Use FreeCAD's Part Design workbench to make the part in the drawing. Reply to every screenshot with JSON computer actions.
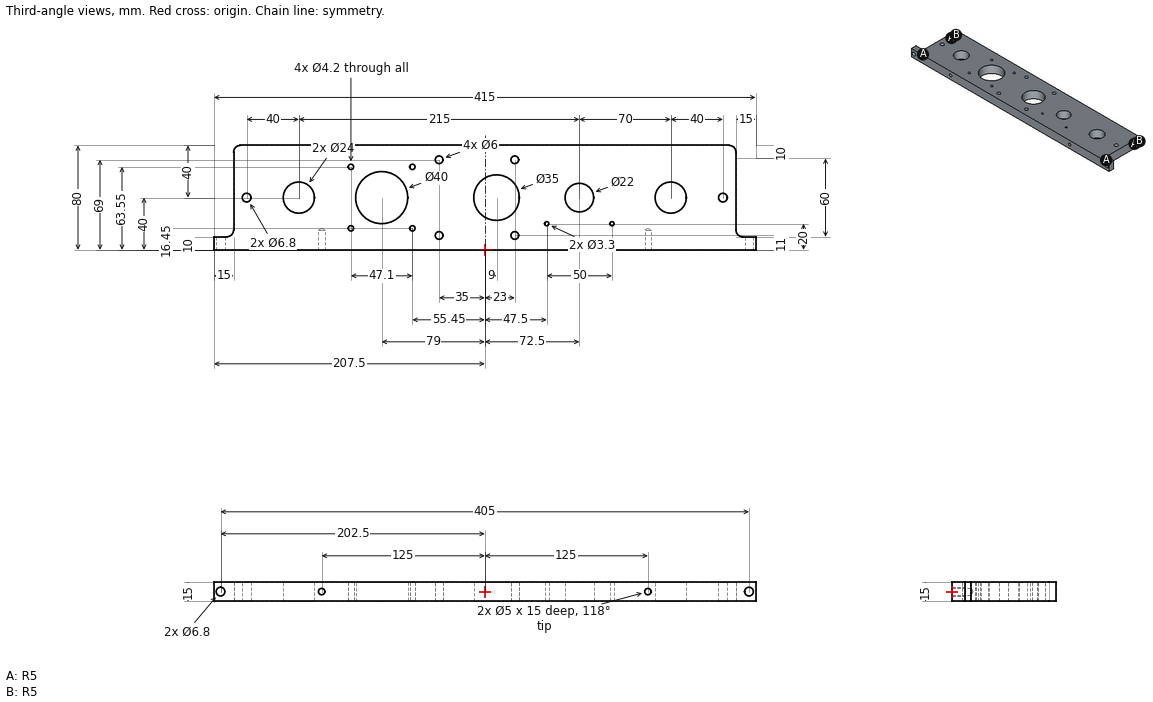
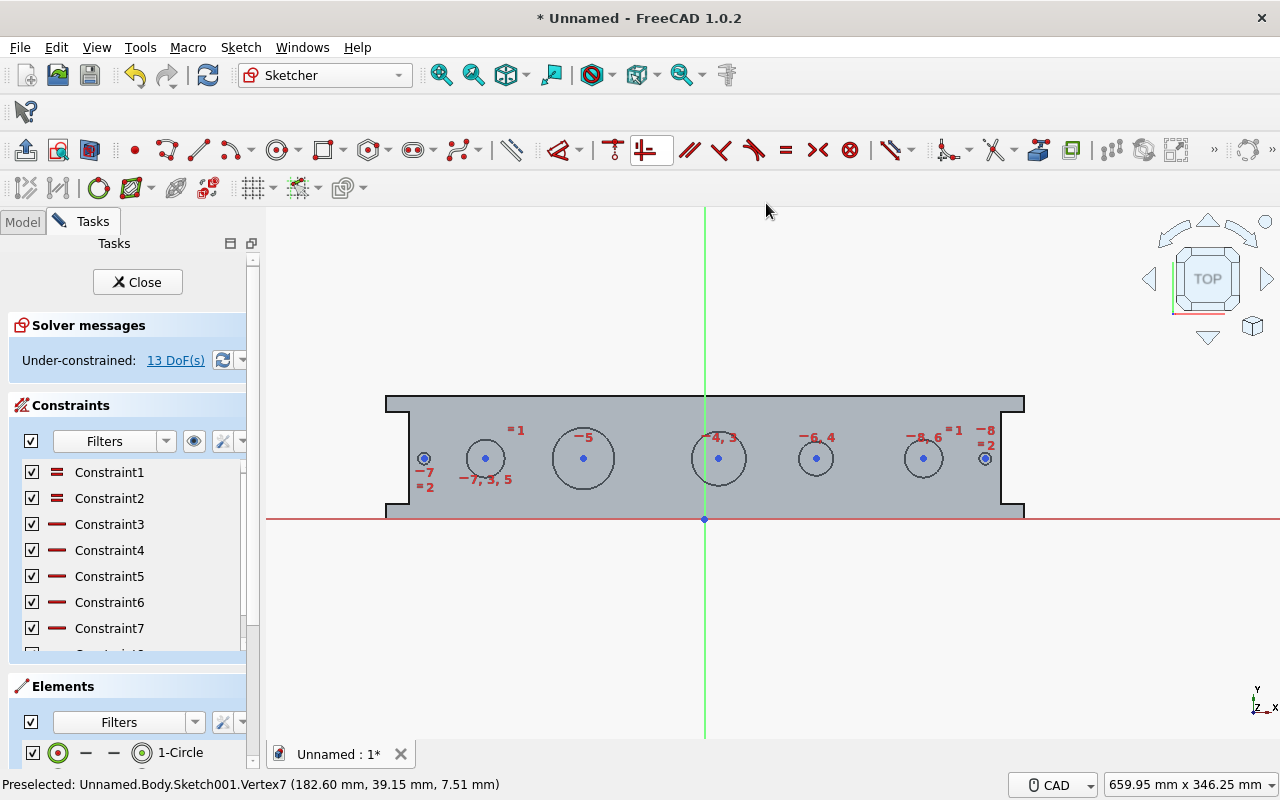
{"action": "left_click", "coordinate": [558, 150]}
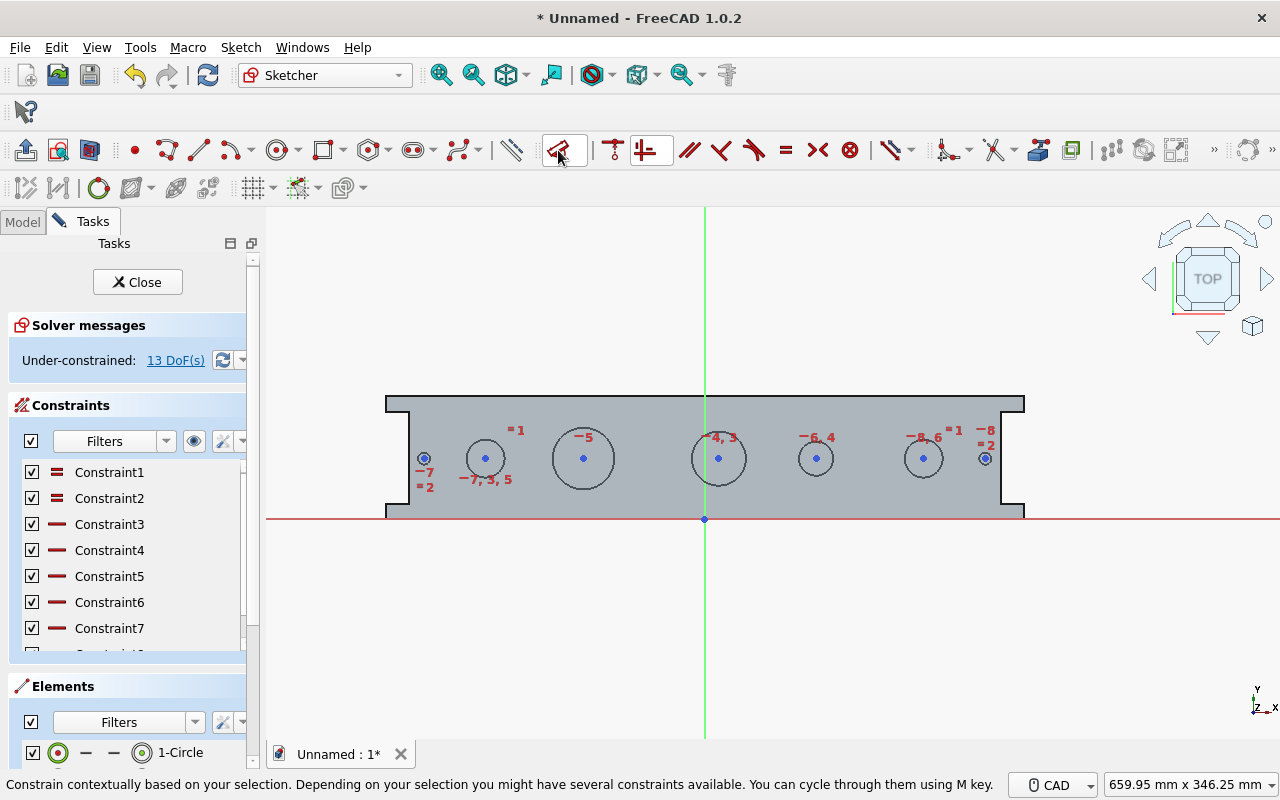
{"action": "left_click", "coordinate": [499, 445]}
{"action": "left_click", "coordinate": [521, 422]}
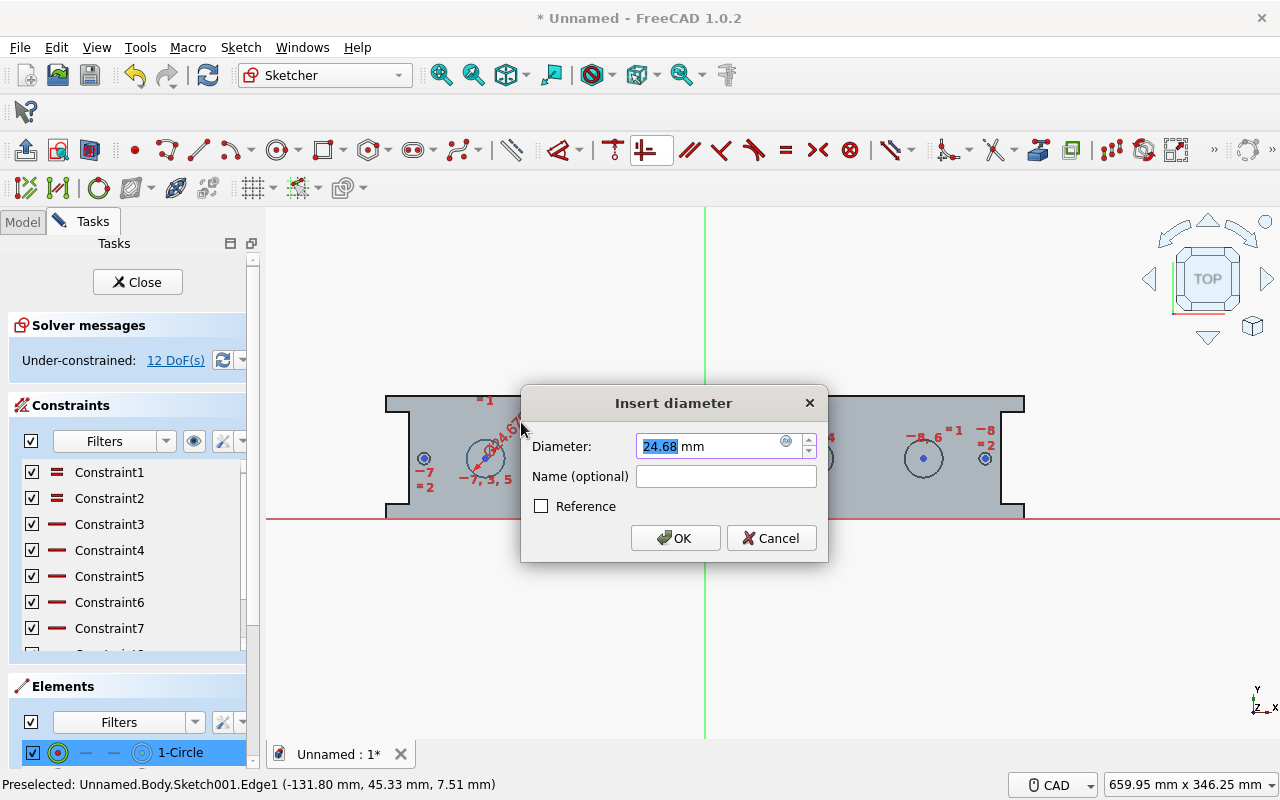
{"action": "type", "text": "24"}
{"action": "key", "text": "Return"}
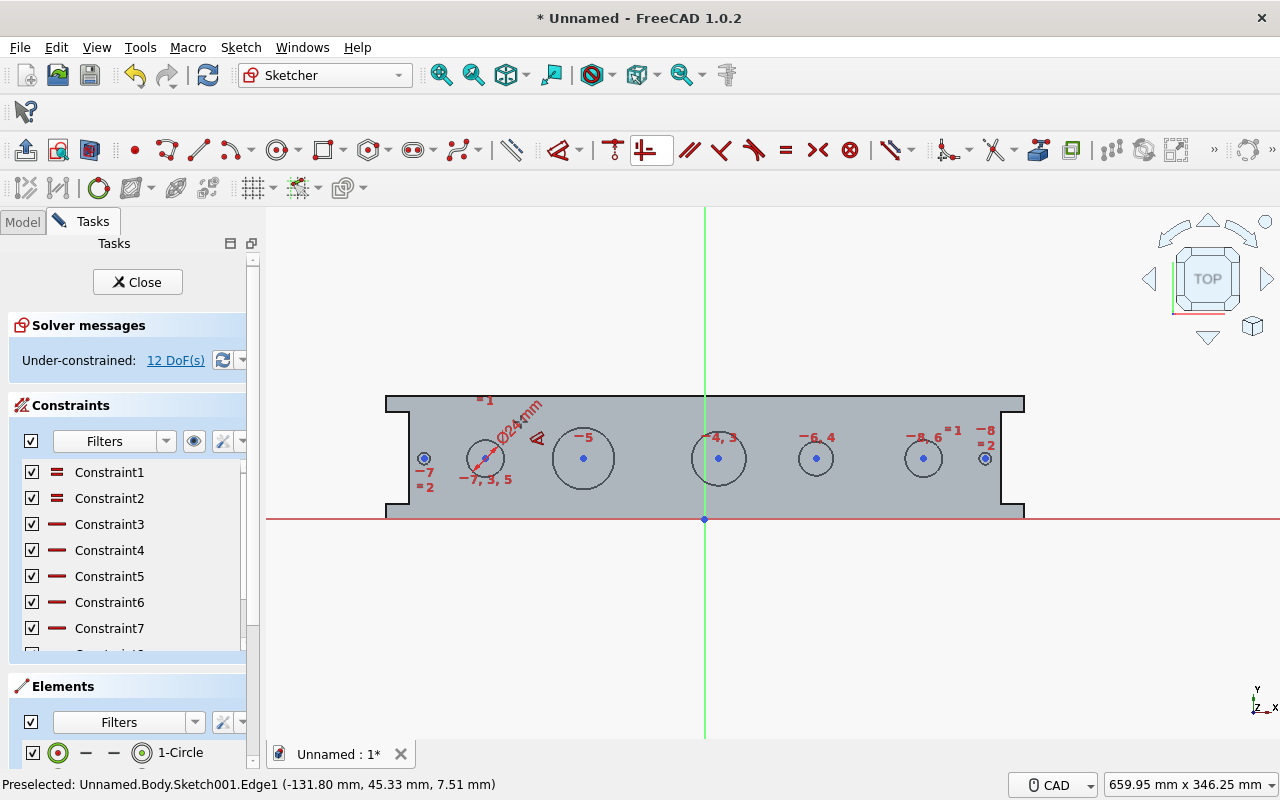
{"action": "left_click", "coordinate": [738, 439]}
{"action": "left_click", "coordinate": [760, 416]}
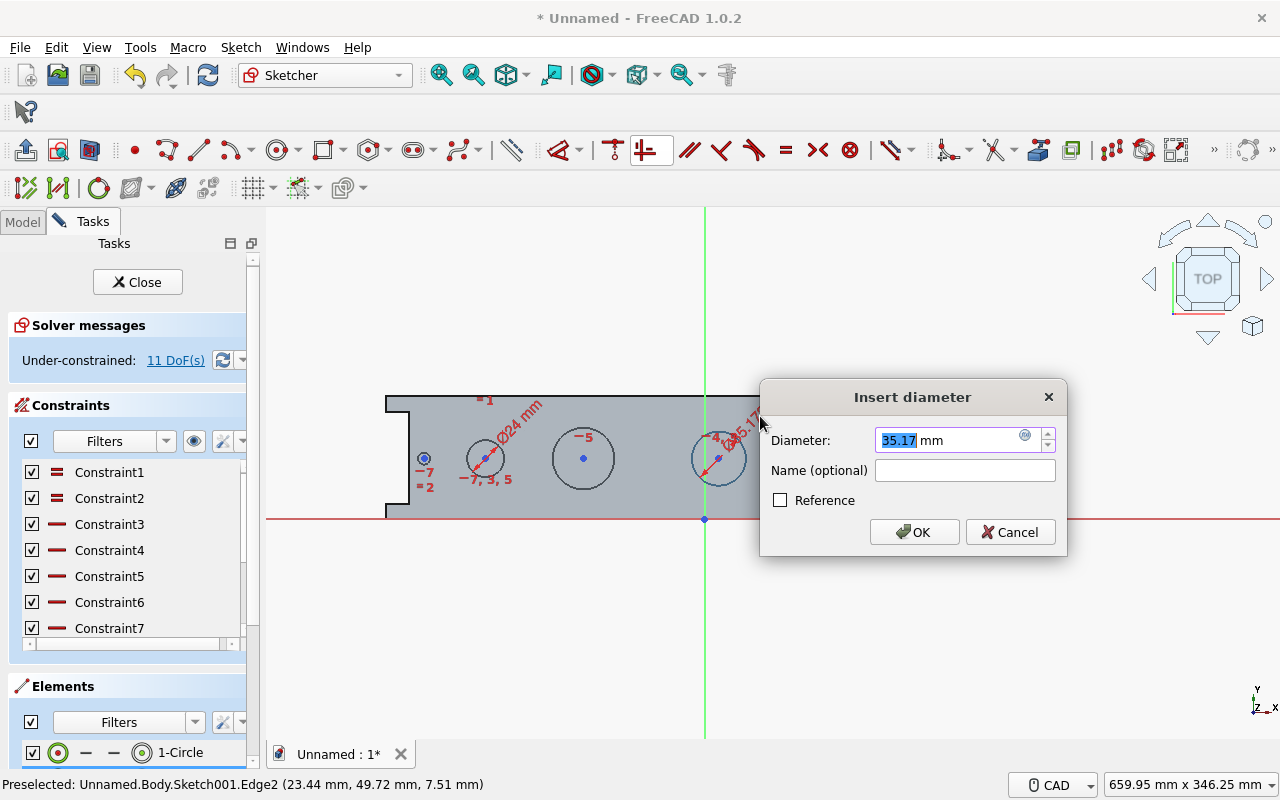
{"action": "type", "text": "35"}
{"action": "key", "text": "Return"}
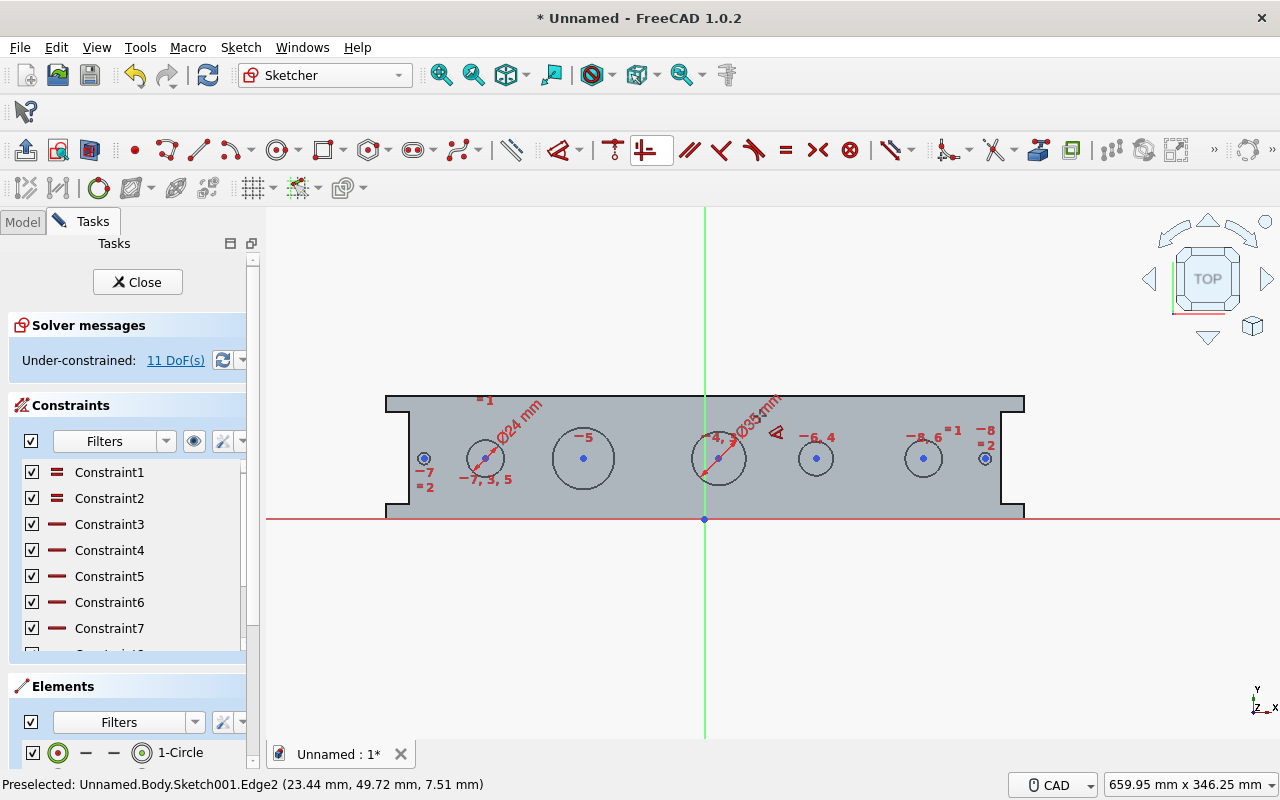
{"action": "left_click", "coordinate": [828, 447]}
{"action": "left_click", "coordinate": [851, 425]}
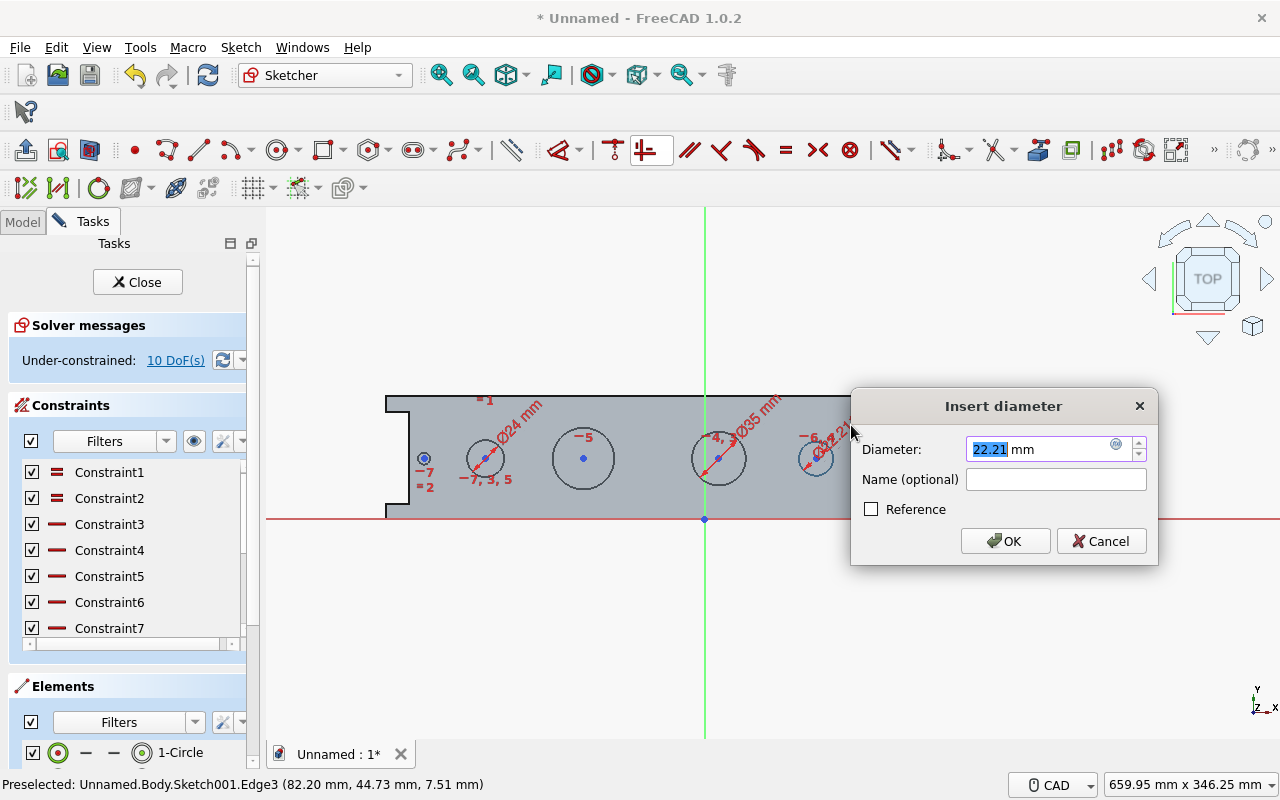
{"action": "type", "text": "22"}
{"action": "key", "text": "Return"}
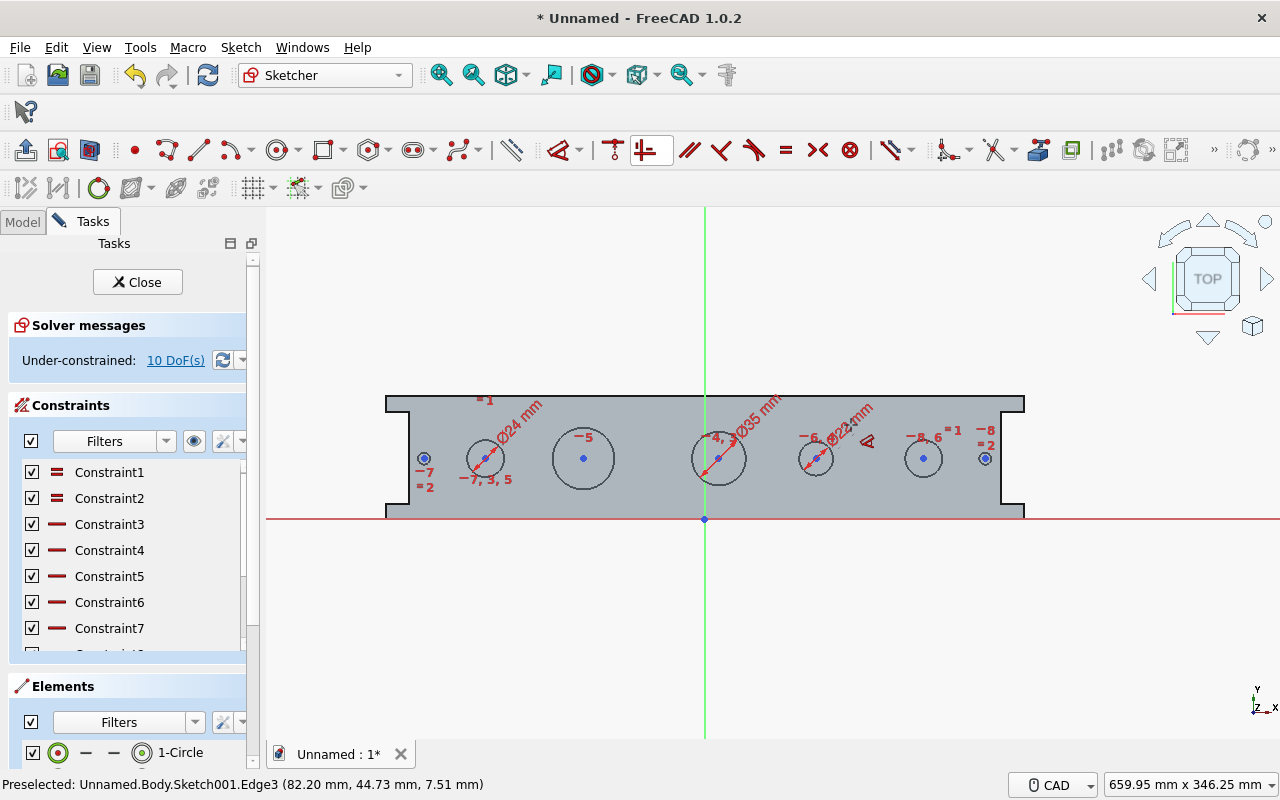
{"action": "left_click", "coordinate": [605, 437]}
{"action": "left_click", "coordinate": [628, 414]}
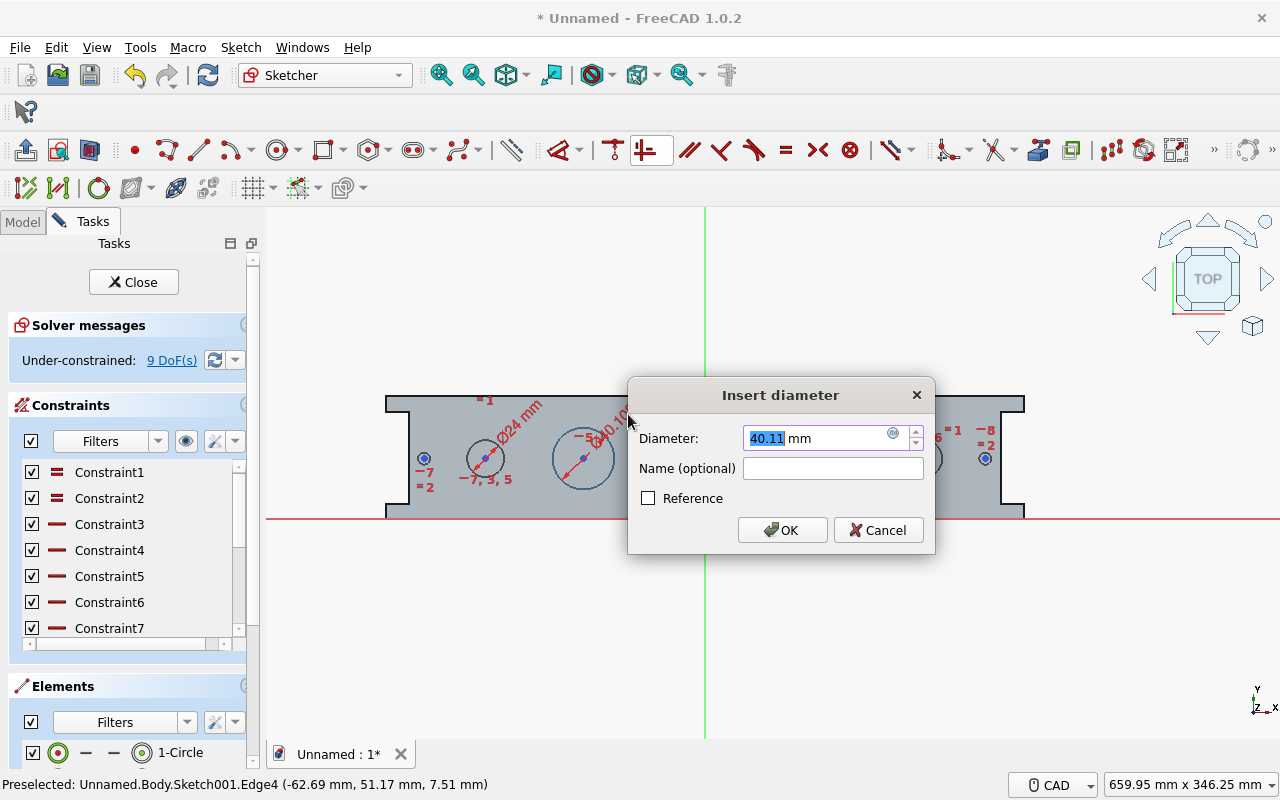
{"action": "type", "text": "40"}
{"action": "key", "text": "Return"}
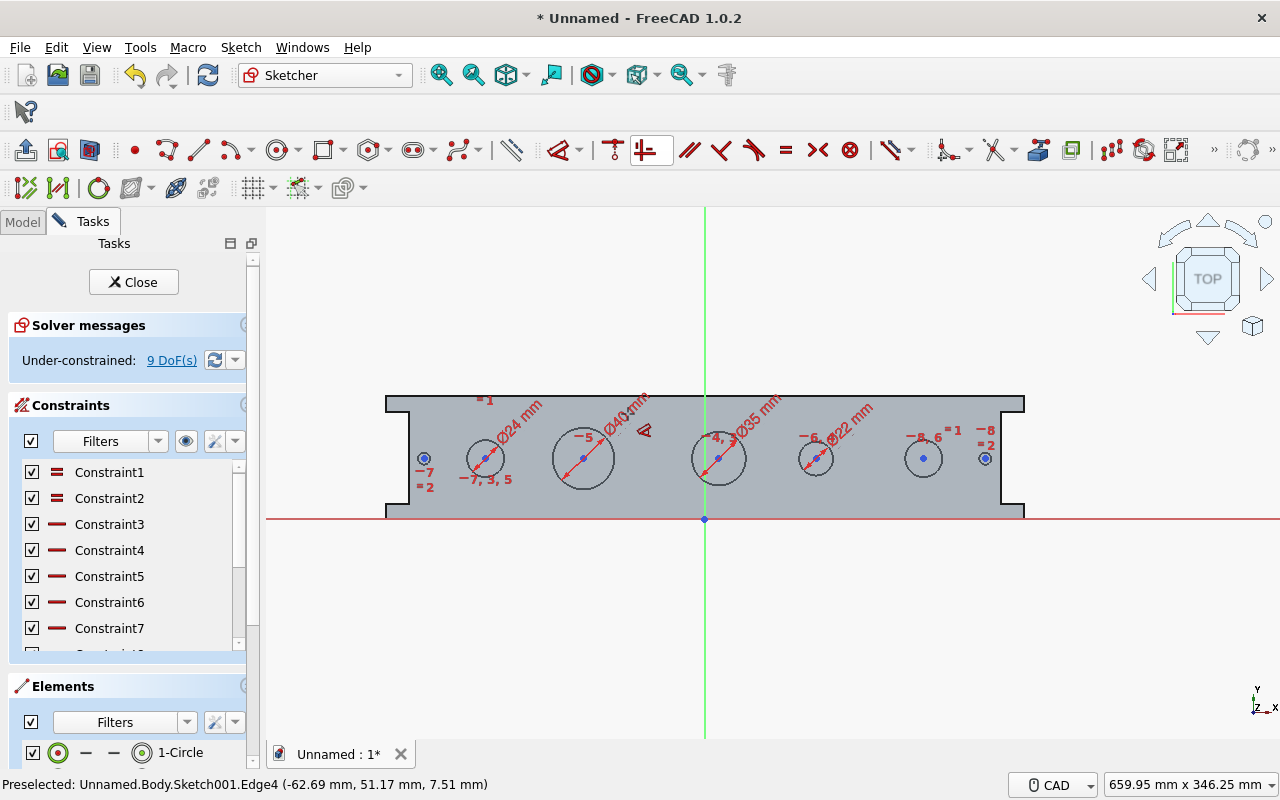
{"action": "scroll", "coordinate": [424, 453], "scroll_direction": "up", "scroll_amount": 7}